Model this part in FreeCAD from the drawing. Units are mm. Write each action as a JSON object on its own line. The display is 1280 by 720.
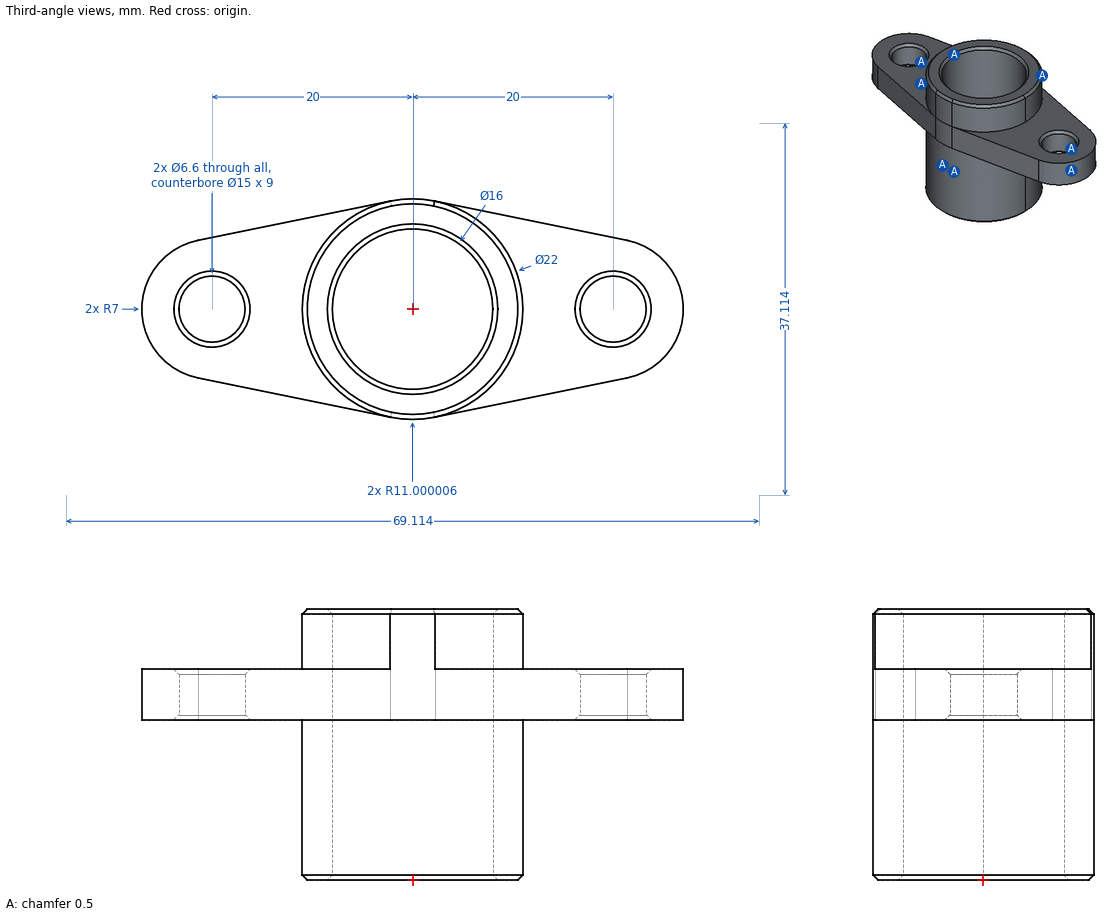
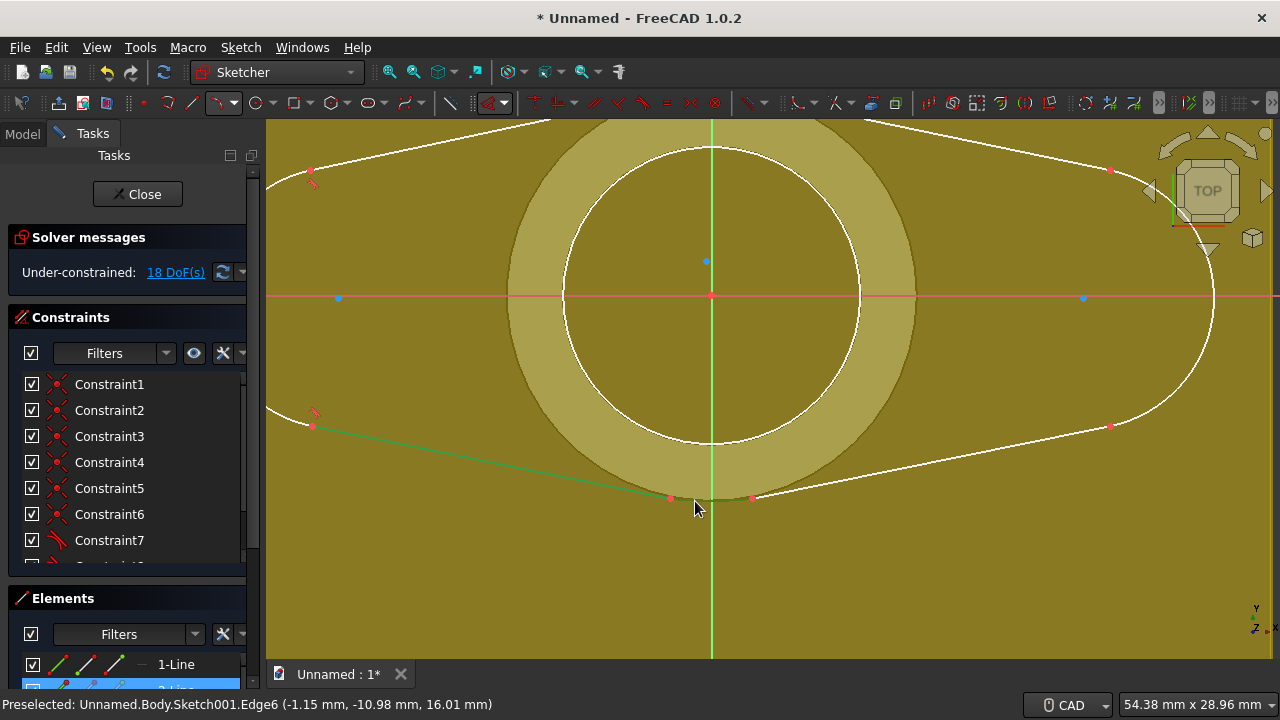
{"action": "left_click", "coordinate": [644, 104]}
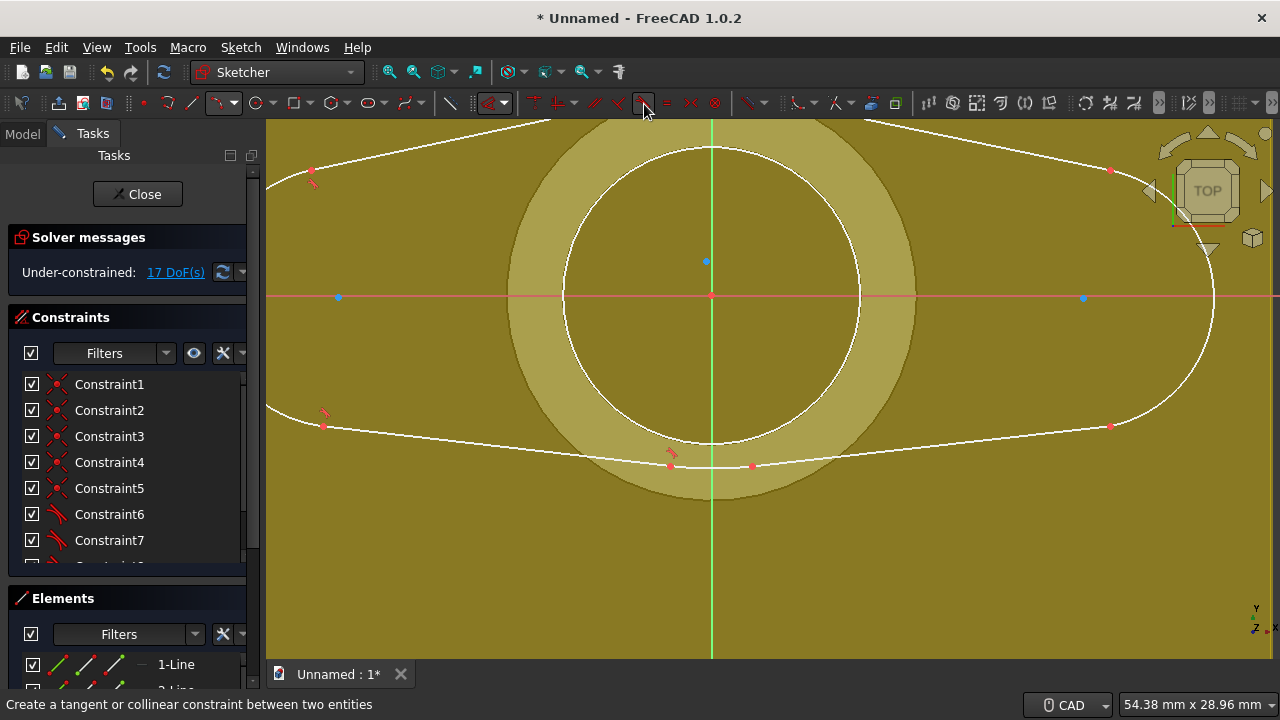
{"action": "left_click", "coordinate": [860, 454]}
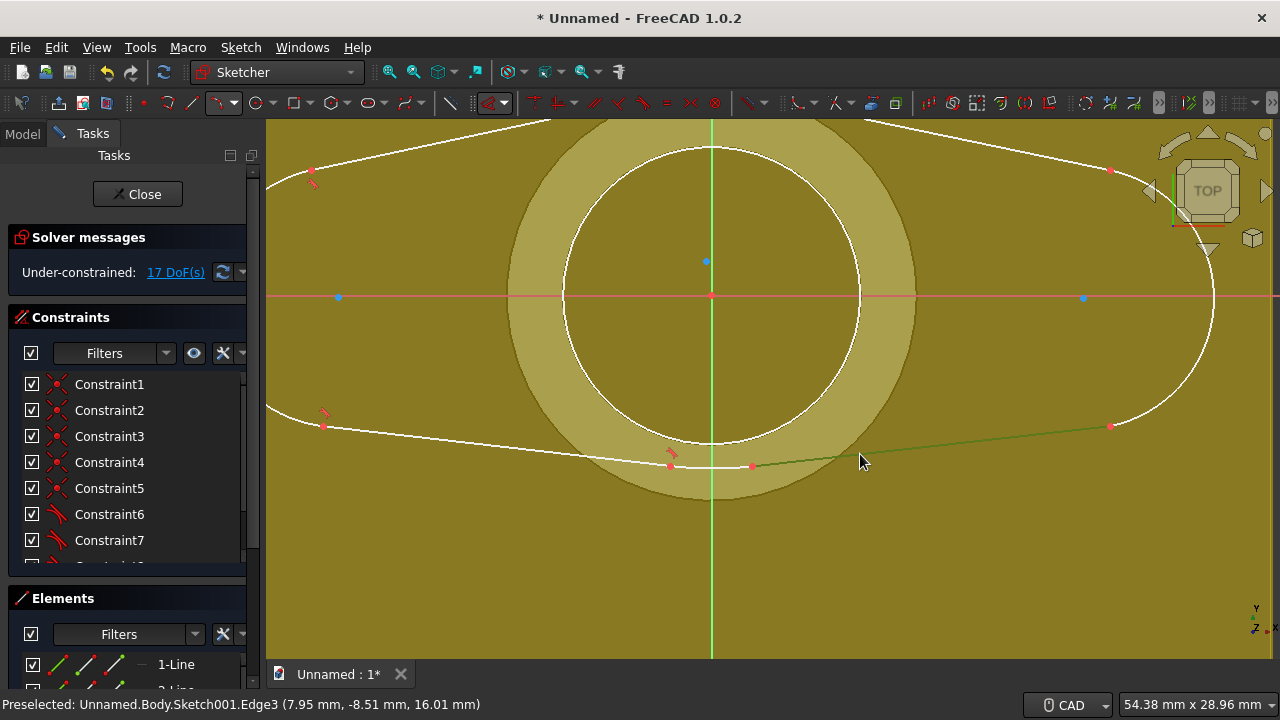
{"action": "left_click", "coordinate": [695, 468]}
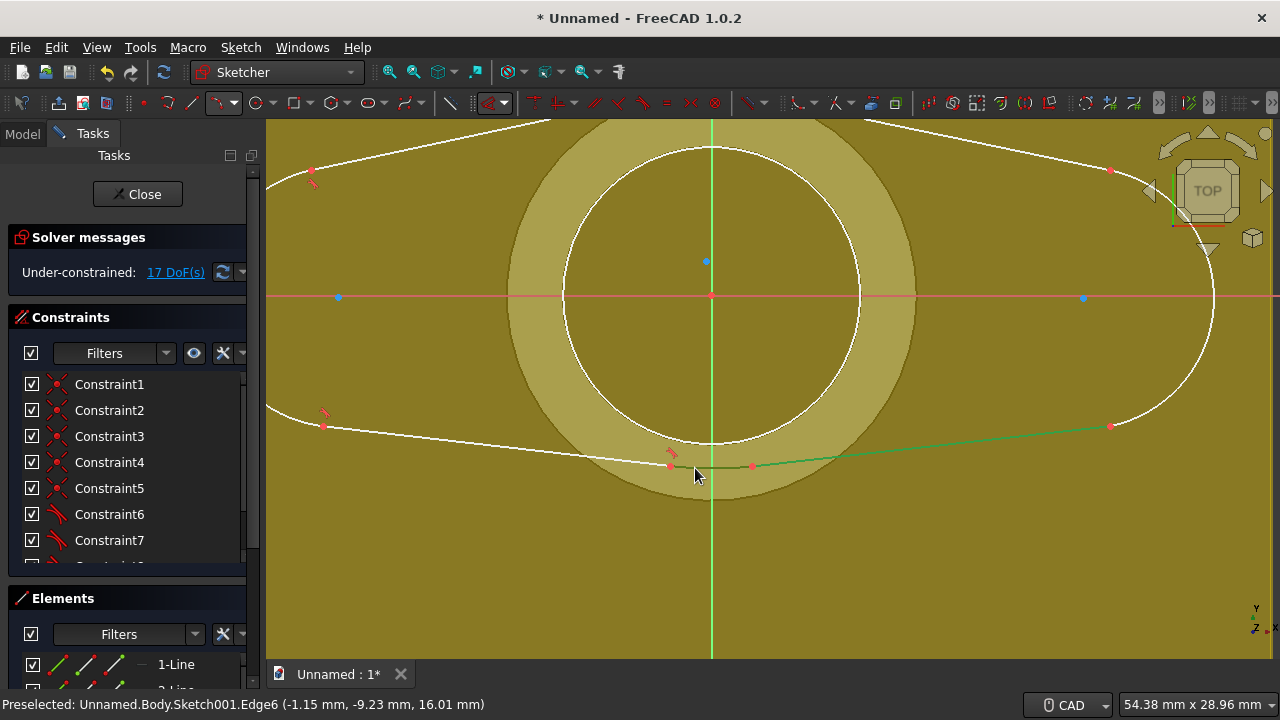
{"action": "left_click", "coordinate": [644, 104]}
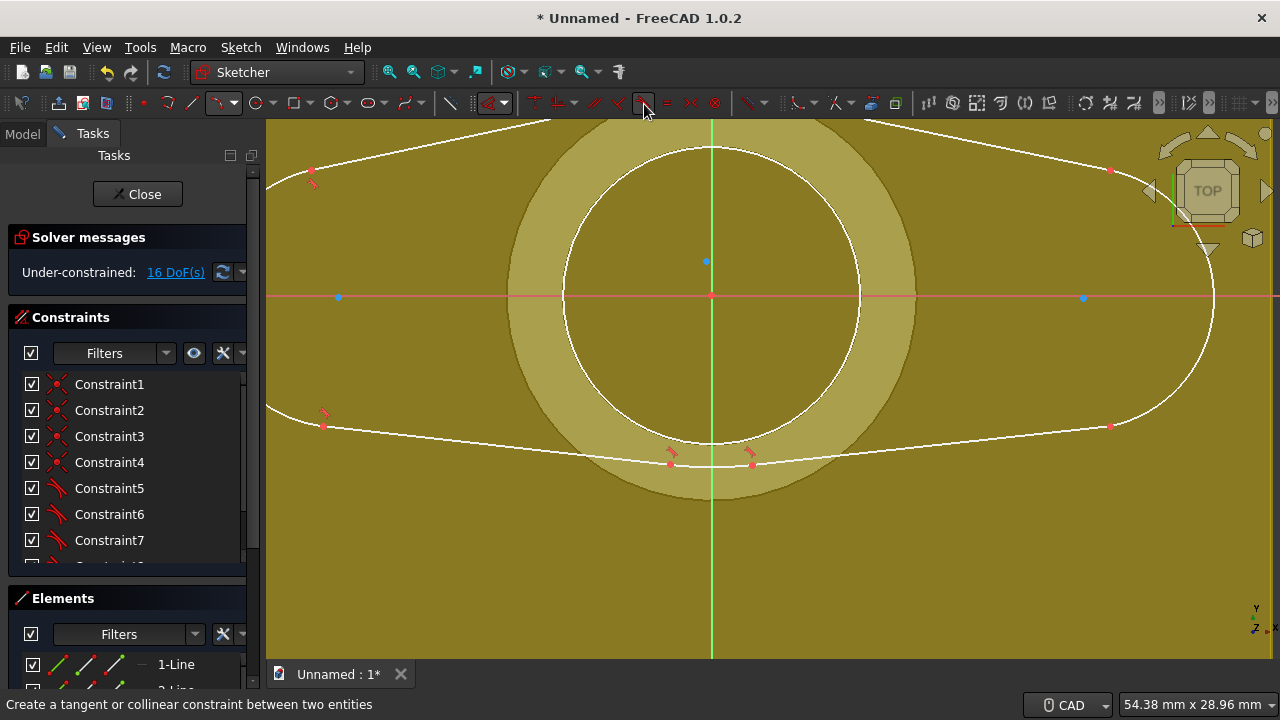
{"action": "left_click", "coordinate": [860, 453]}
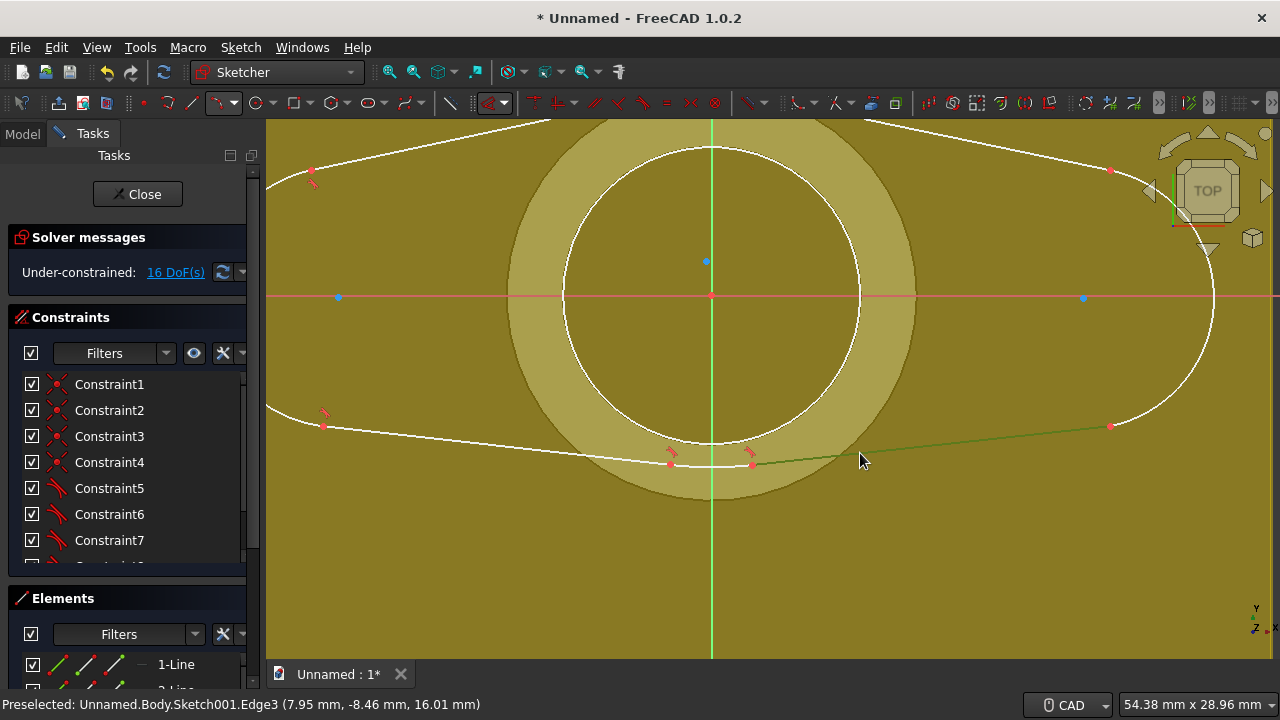
{"action": "scroll", "coordinate": [696, 503], "scroll_direction": "down", "scroll_amount": 3}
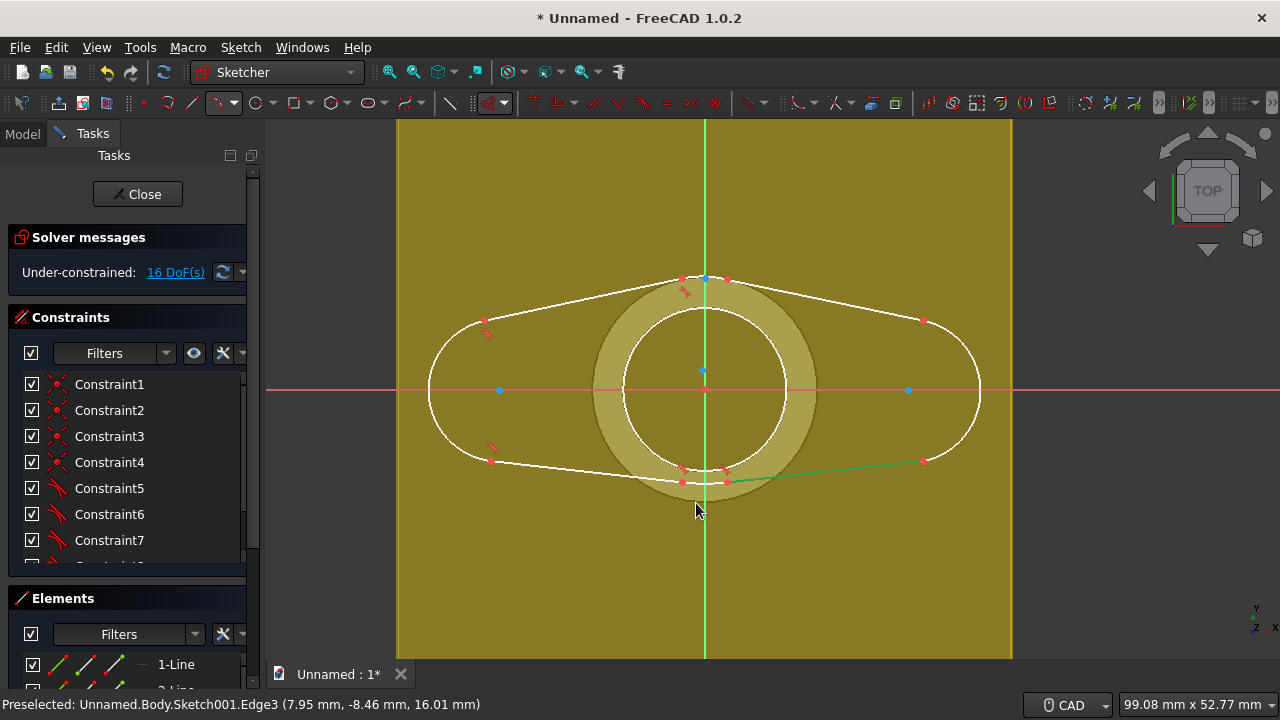
{"action": "left_click", "coordinate": [970, 428]}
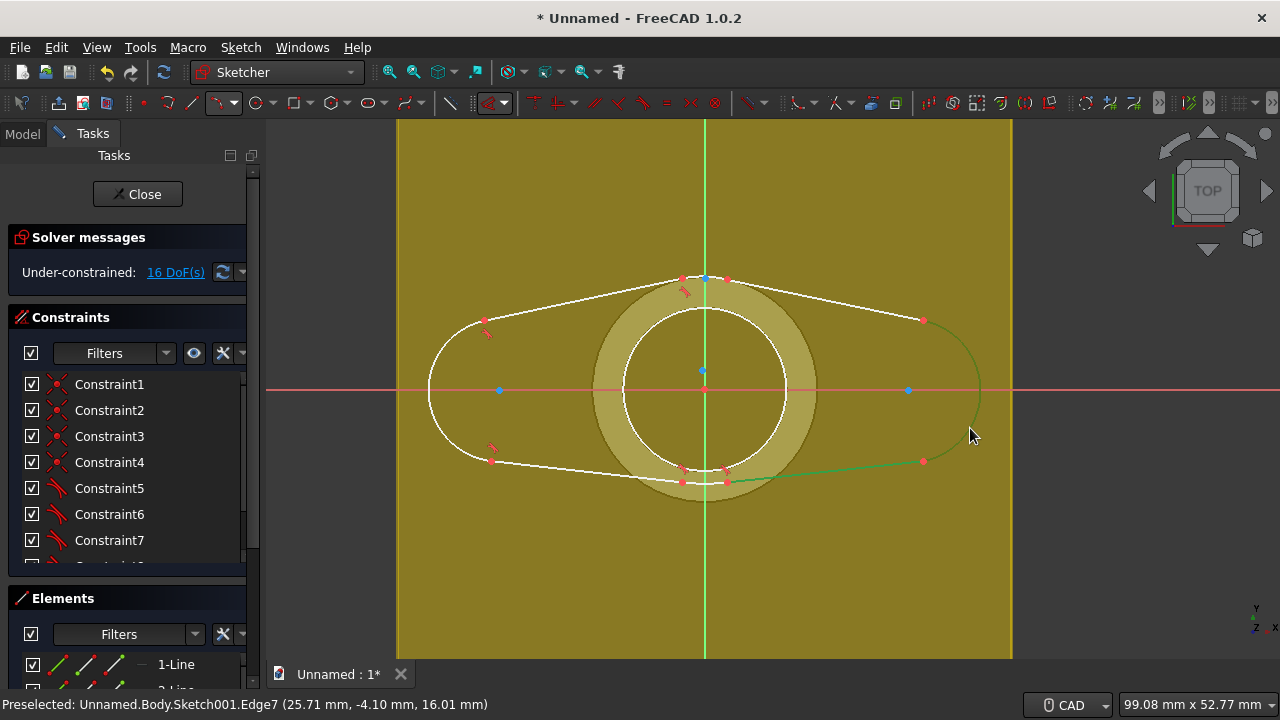
{"action": "key", "text": "t"}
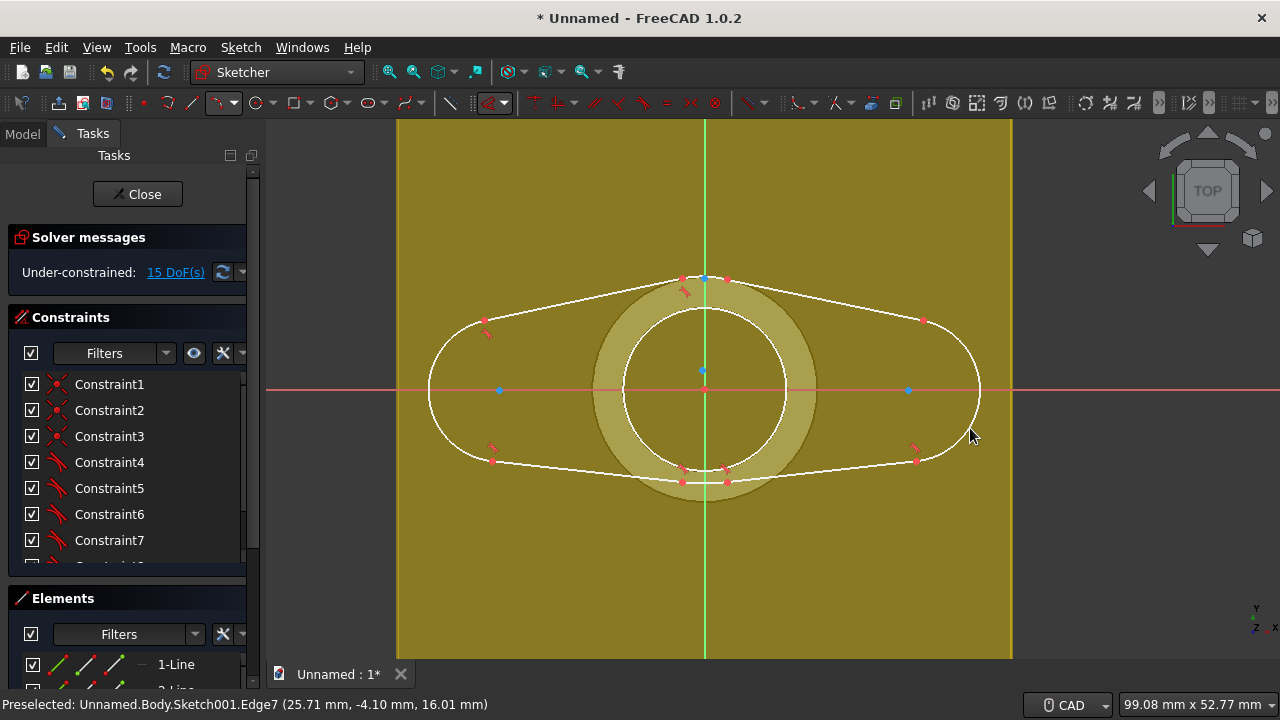
{"action": "left_click", "coordinate": [865, 308]}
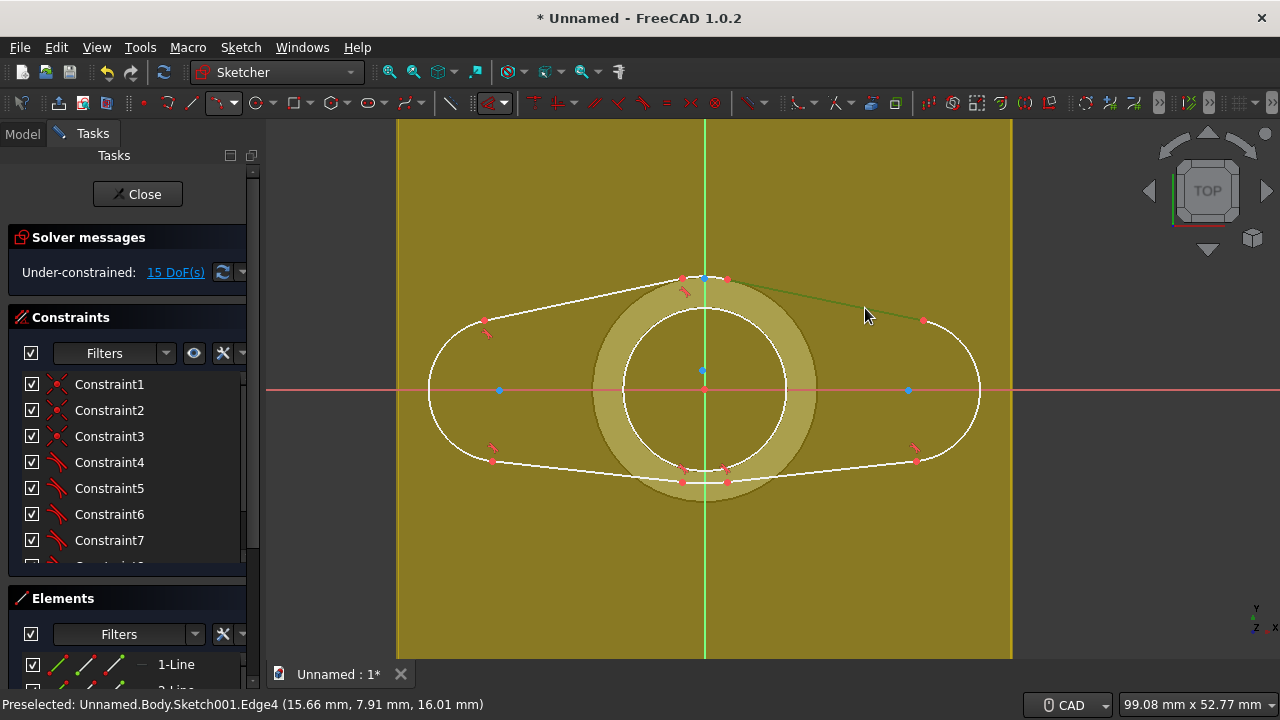
{"action": "left_click", "coordinate": [967, 431]}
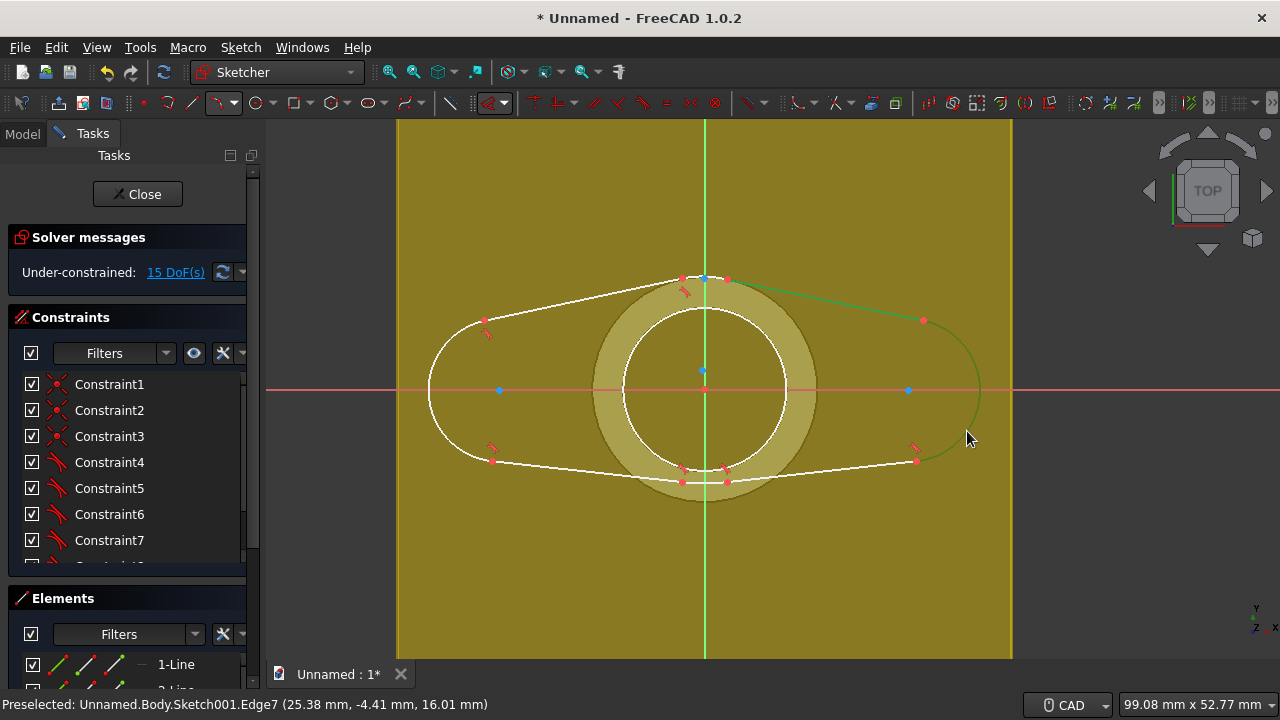
{"action": "left_click", "coordinate": [644, 104]}